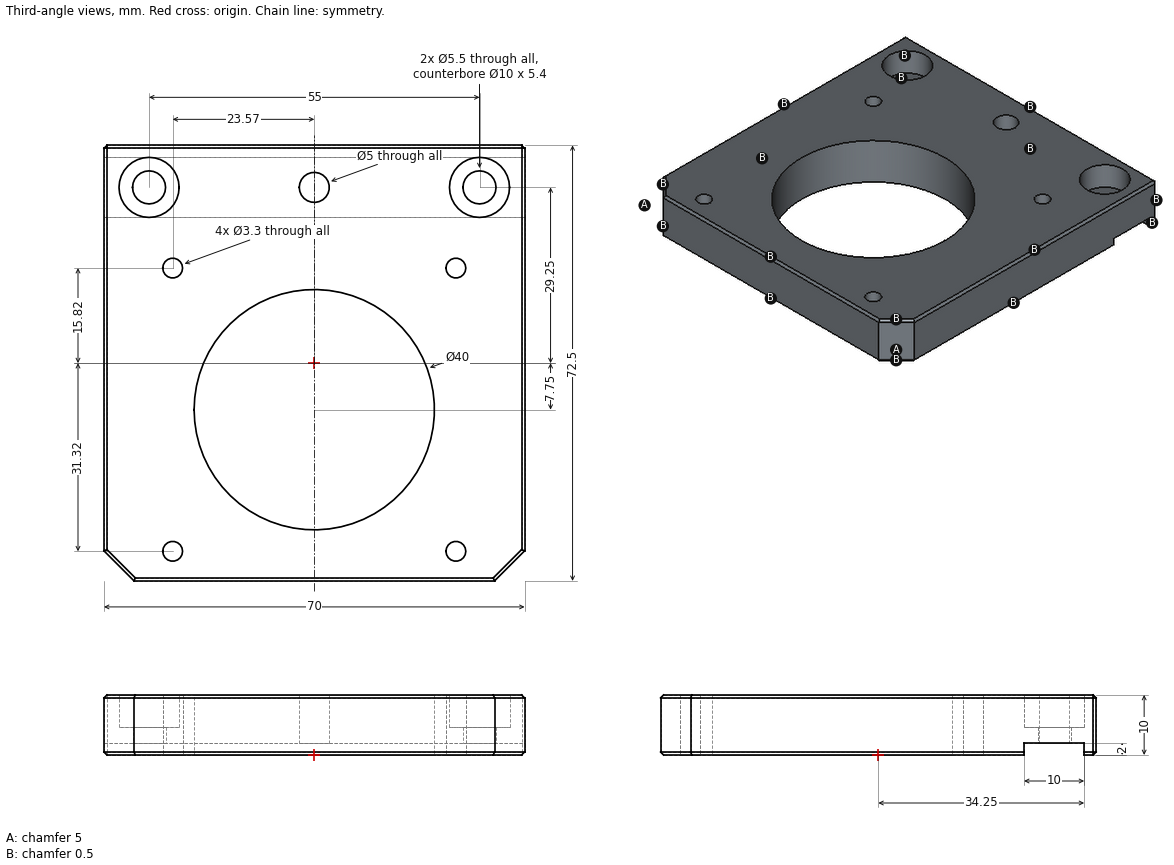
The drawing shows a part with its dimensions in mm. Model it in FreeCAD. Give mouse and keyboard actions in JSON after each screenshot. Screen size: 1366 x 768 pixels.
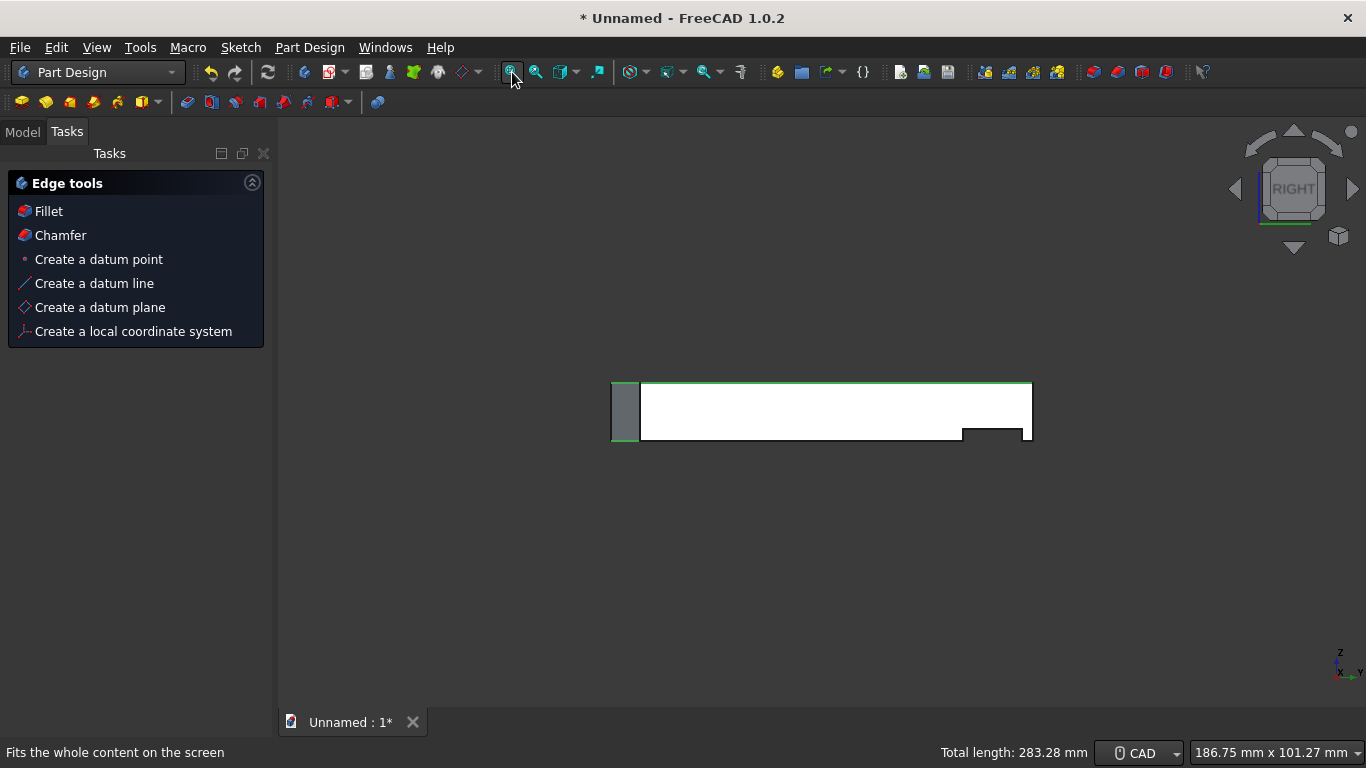
{"action": "left_click", "coordinate": [802, 440], "text": "ctrl"}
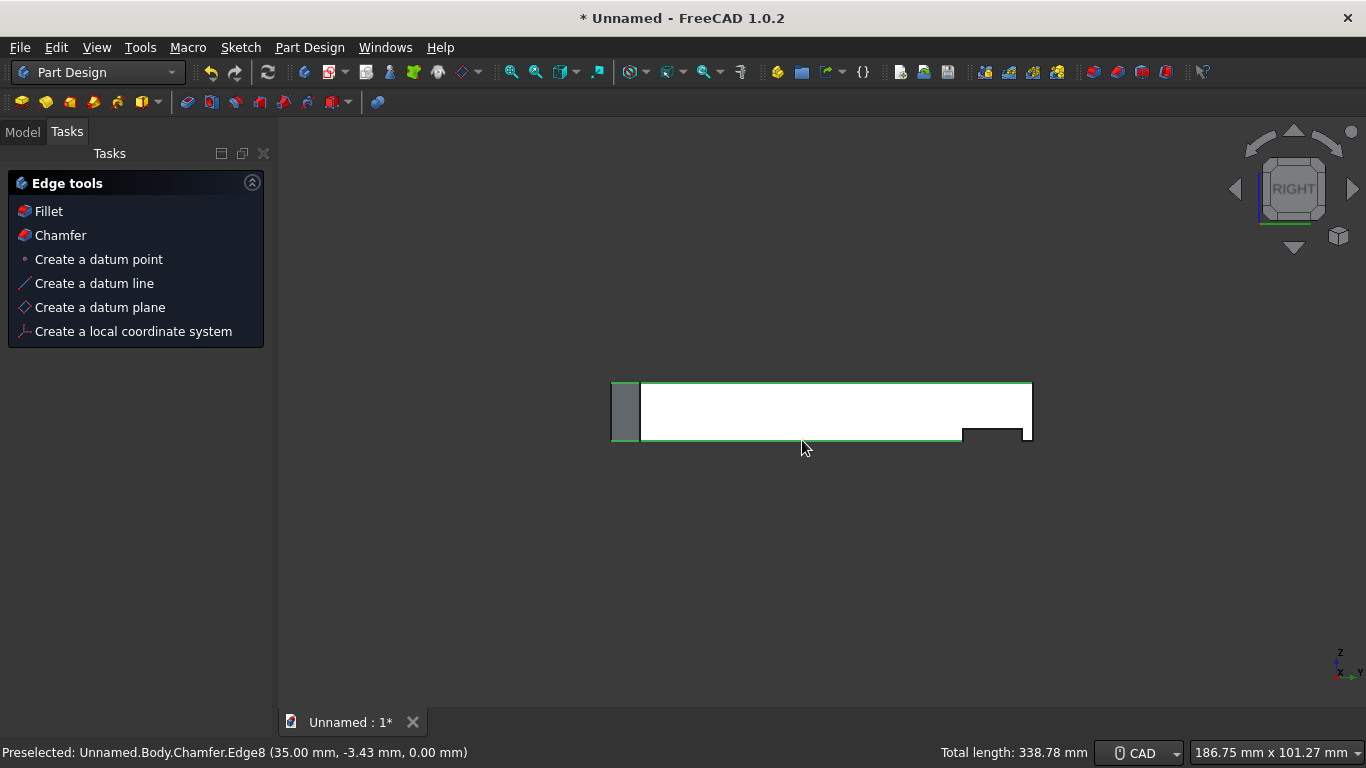
{"action": "key", "text": "5"}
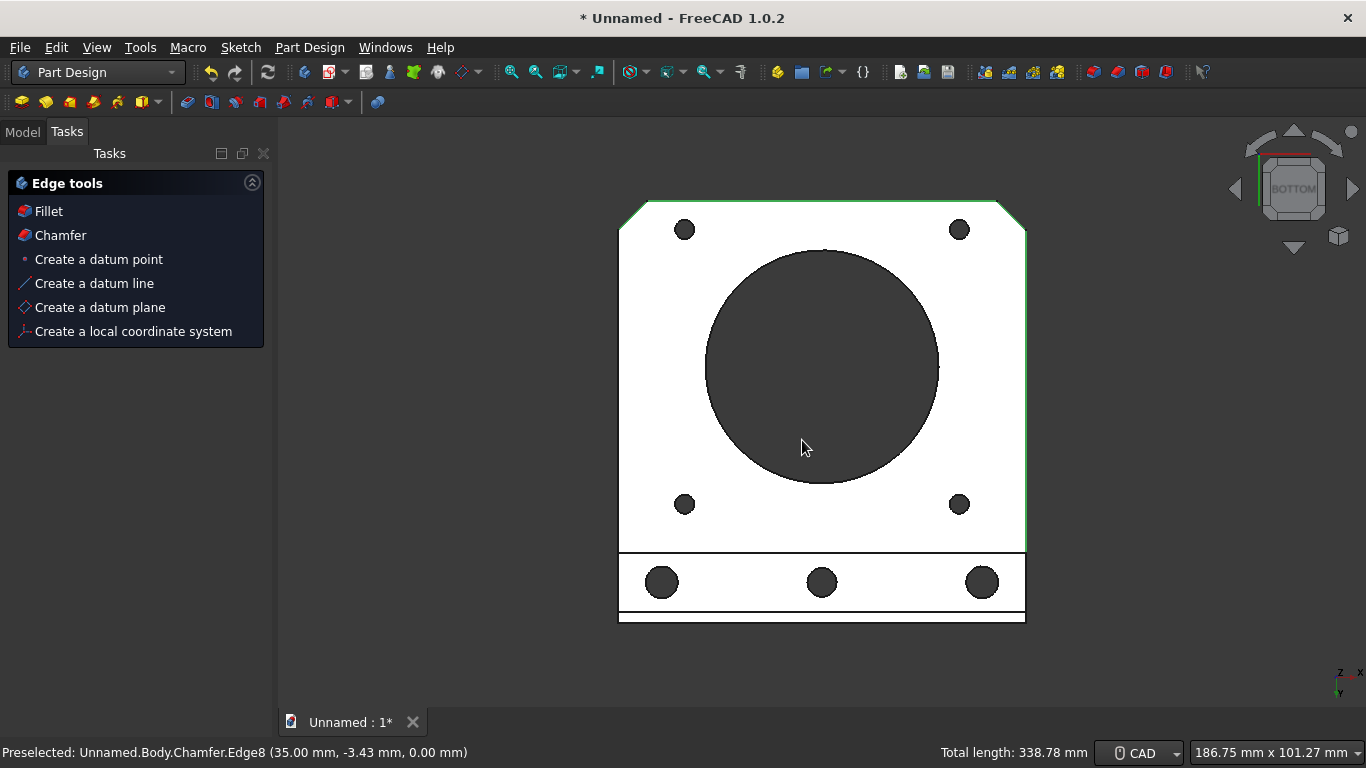
{"action": "left_click", "coordinate": [618, 391], "text": "ctrl"}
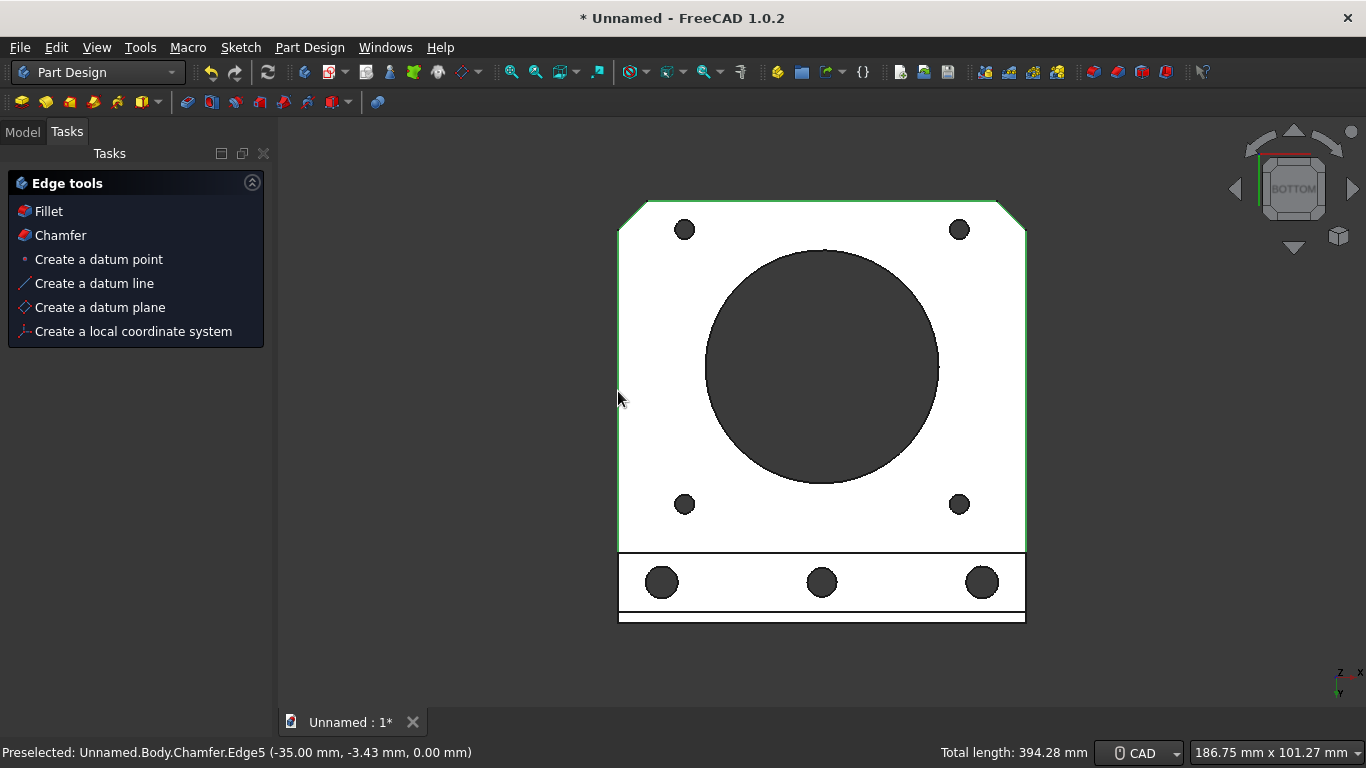
{"action": "key", "text": "4"}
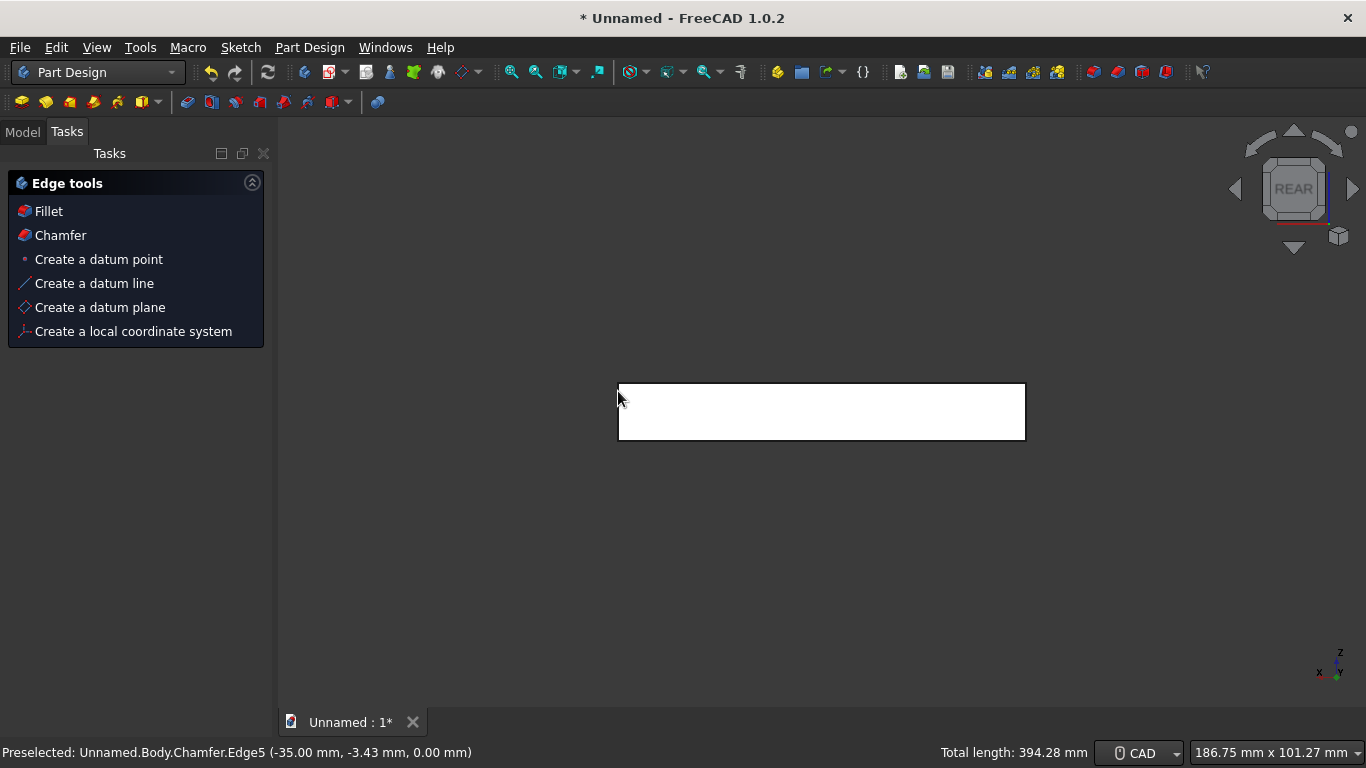
{"action": "left_click", "coordinate": [512, 72]}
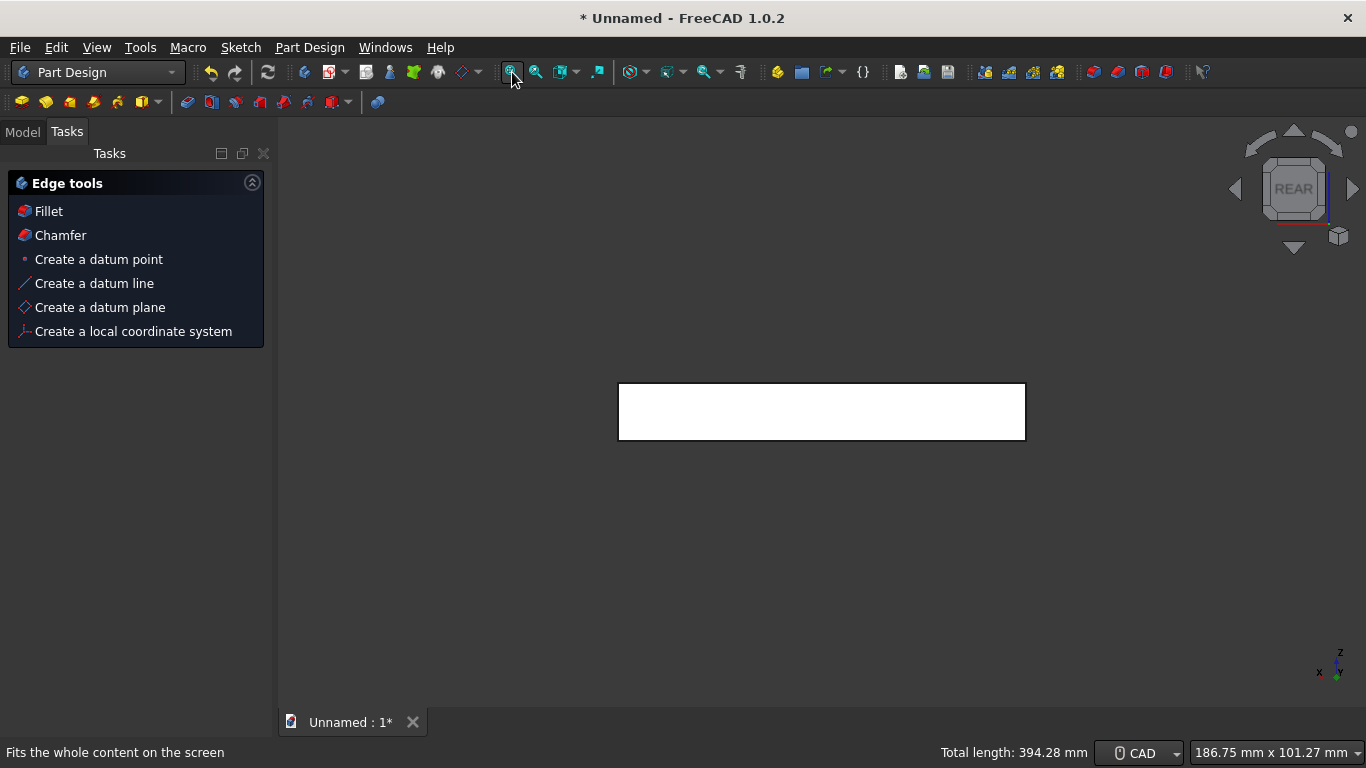
{"action": "left_click", "coordinate": [647, 411], "text": "ctrl"}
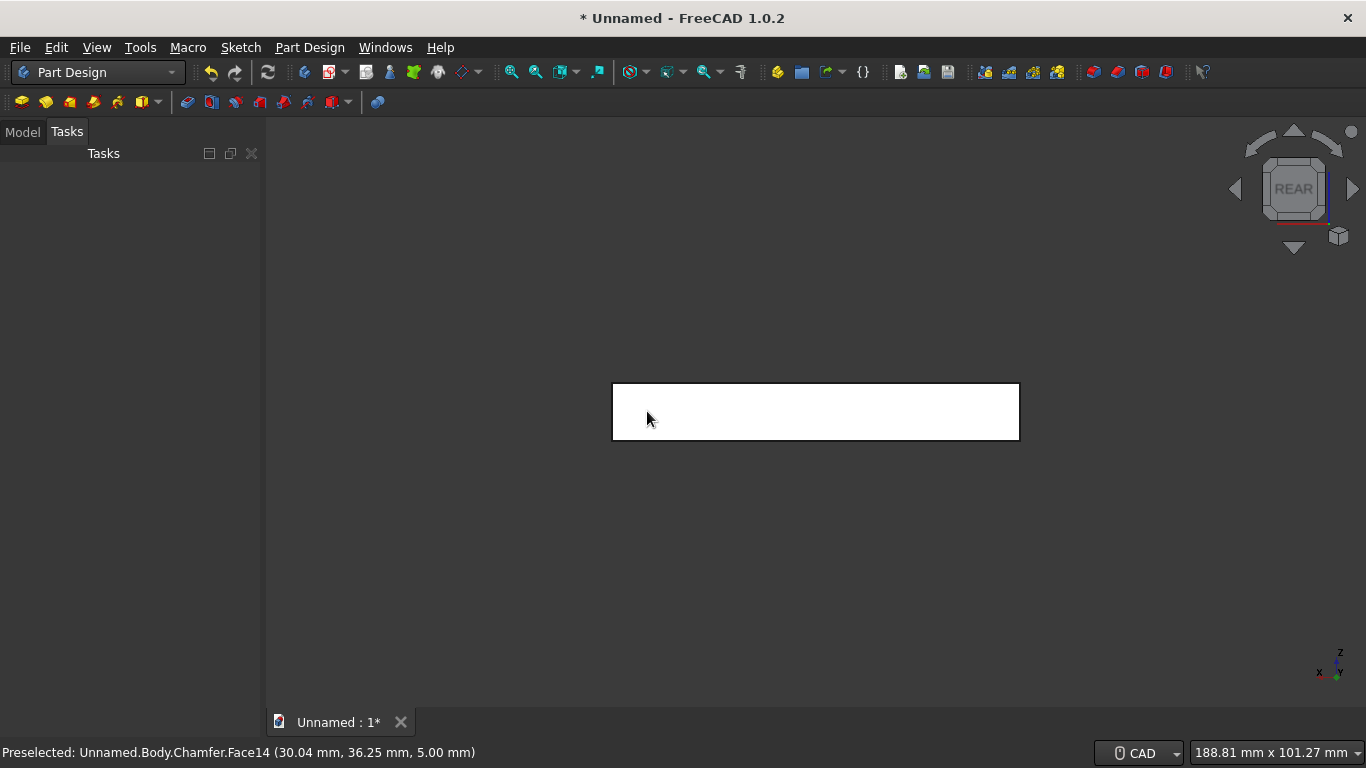
{"action": "scroll", "coordinate": [612, 440], "scroll_direction": "up", "scroll_amount": 7}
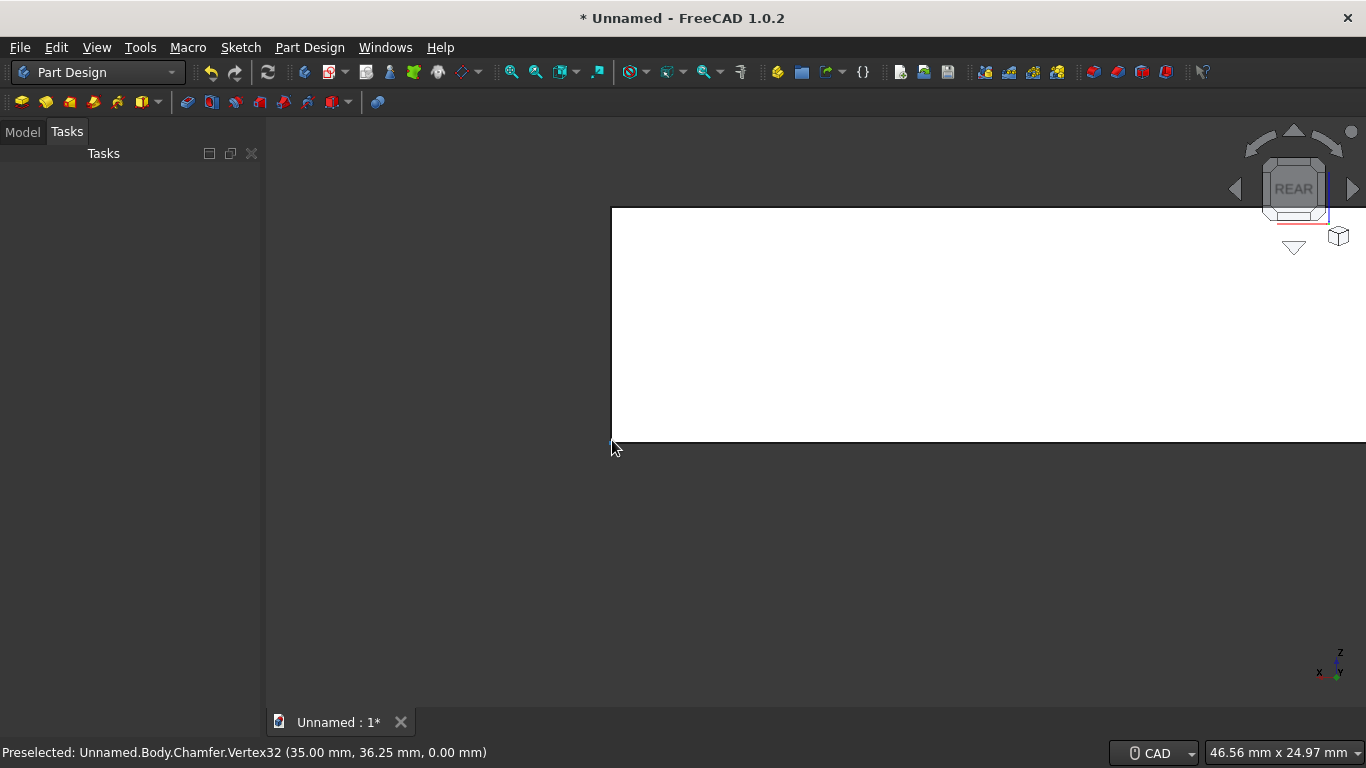
{"action": "key", "text": "v f"}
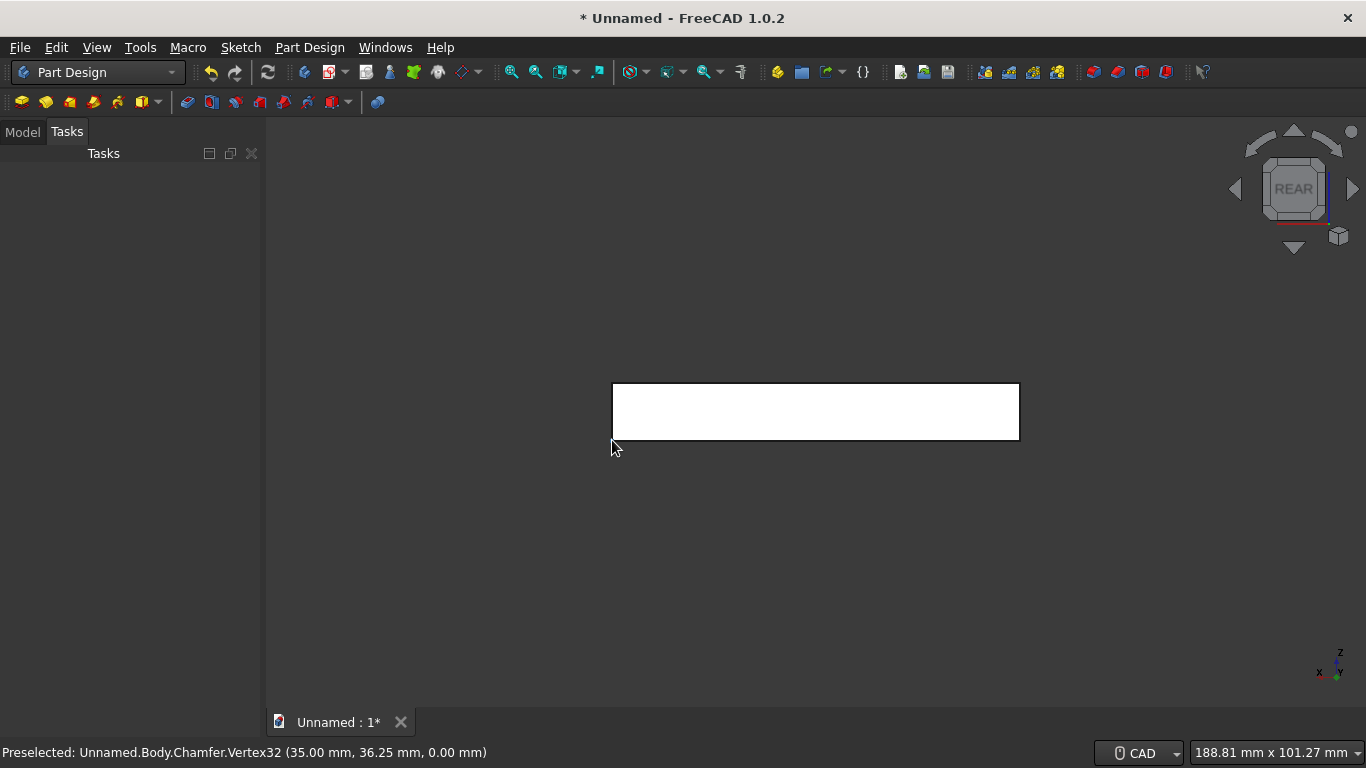
{"action": "key", "text": "6"}